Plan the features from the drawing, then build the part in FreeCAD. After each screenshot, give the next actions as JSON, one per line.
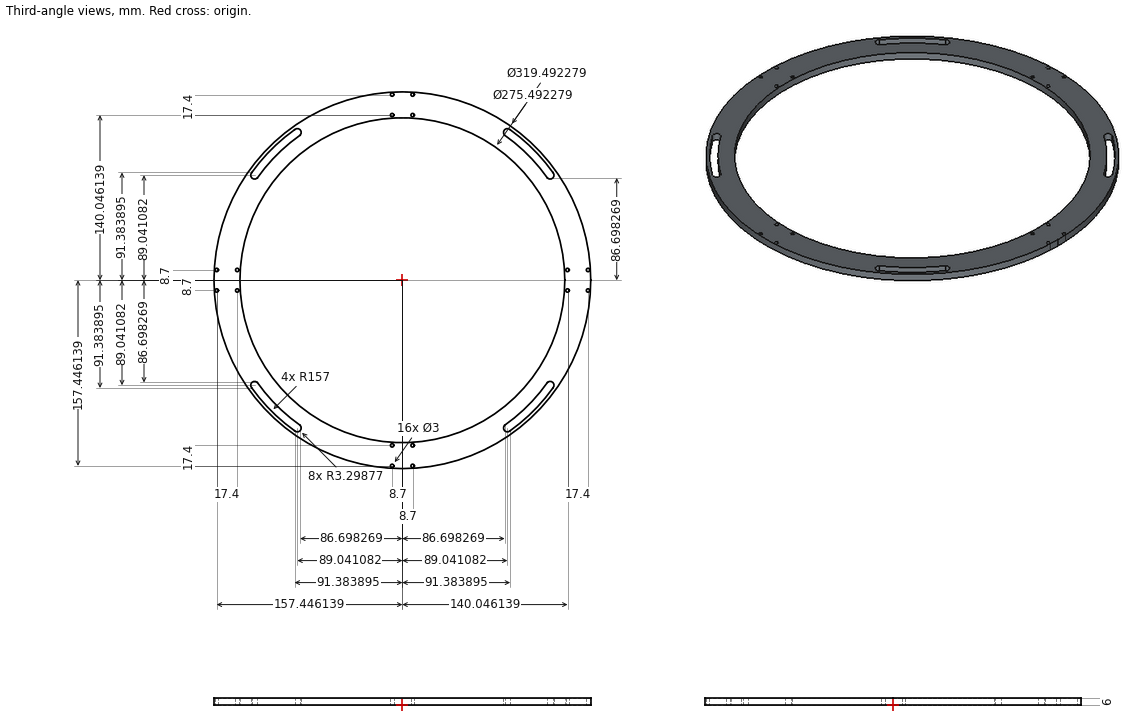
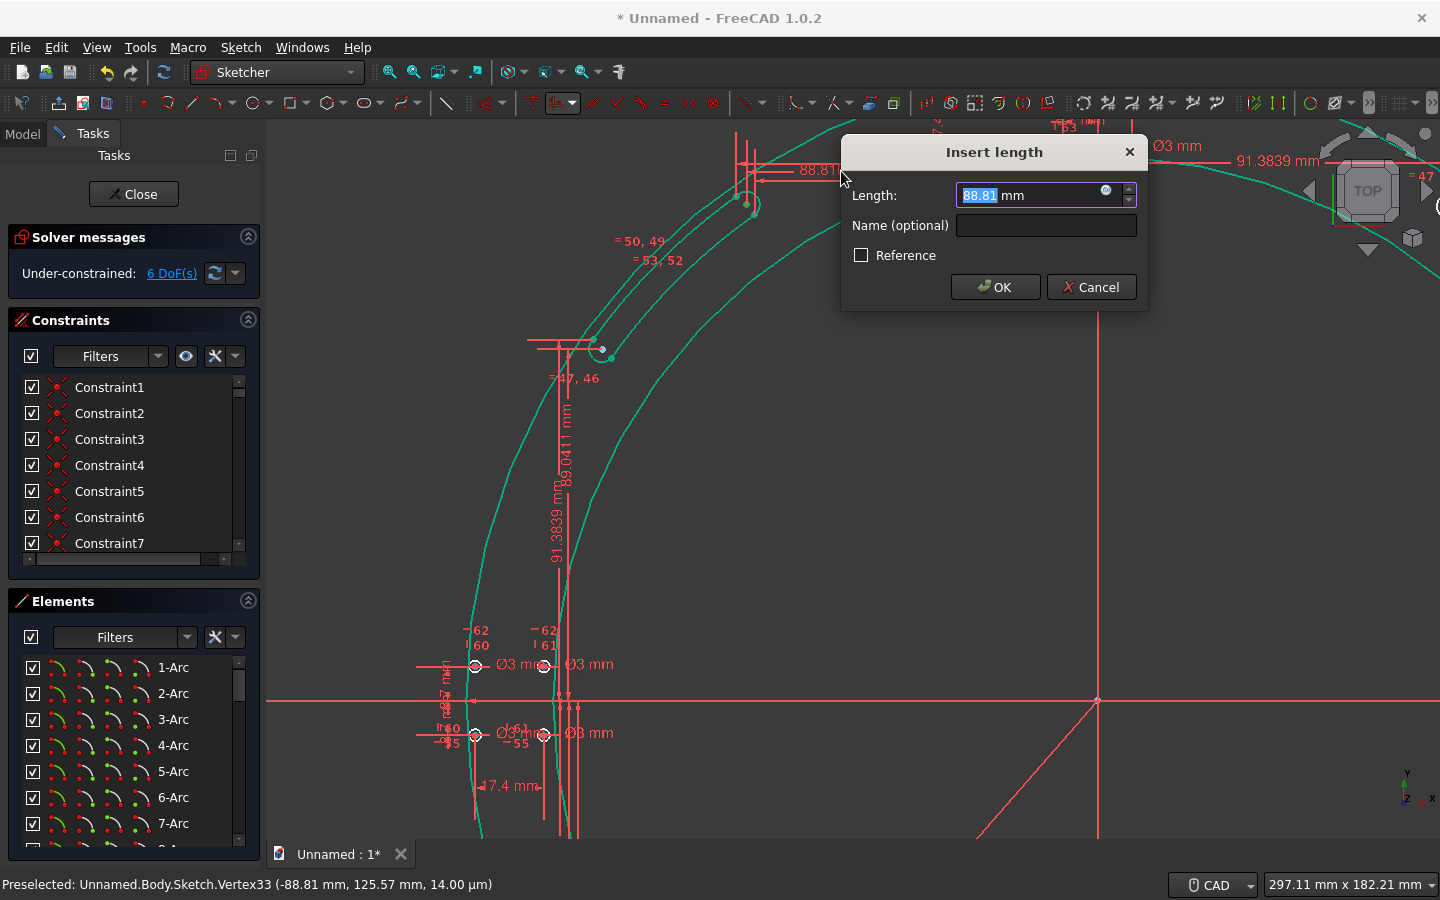
{"action": "type", "text": "89.041082"}
{"action": "key", "text": "Return"}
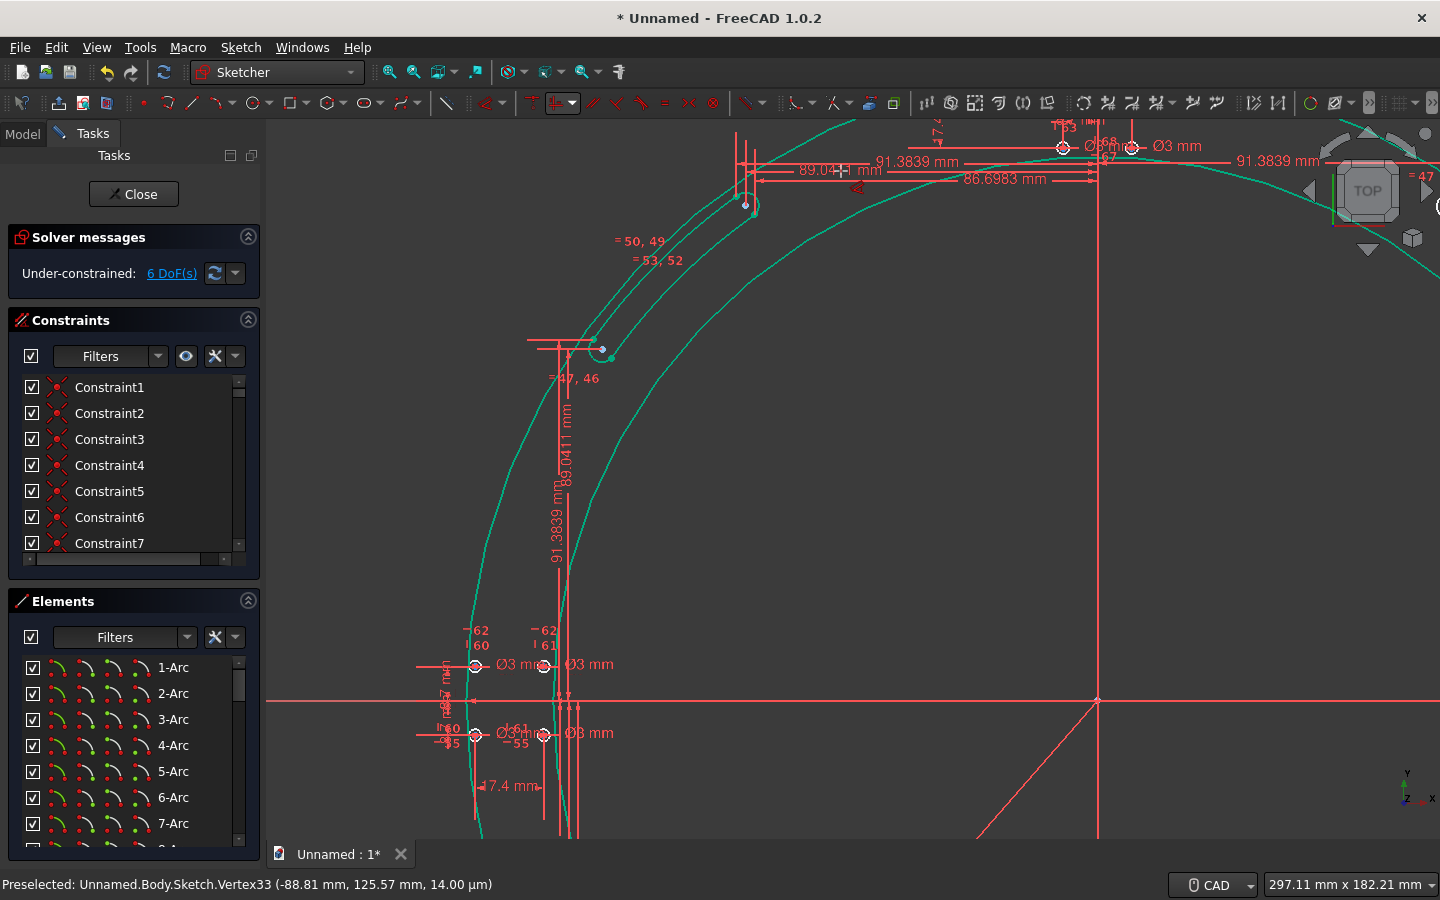
{"action": "scroll", "coordinate": [602, 350], "scroll_direction": "down", "scroll_amount": 5}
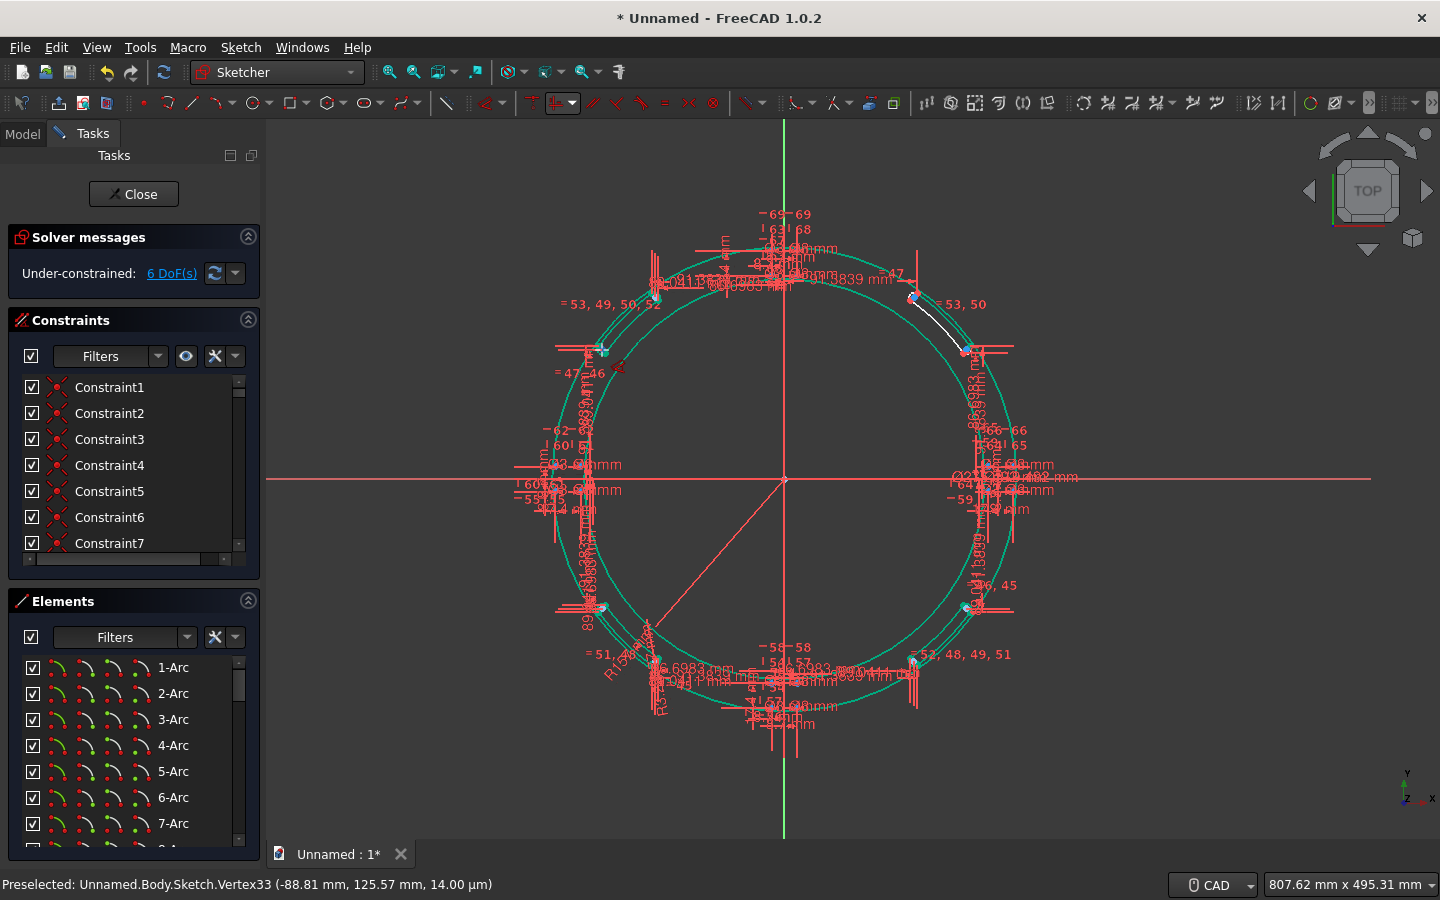
{"action": "scroll", "coordinate": [914, 297], "scroll_direction": "up", "scroll_amount": 5}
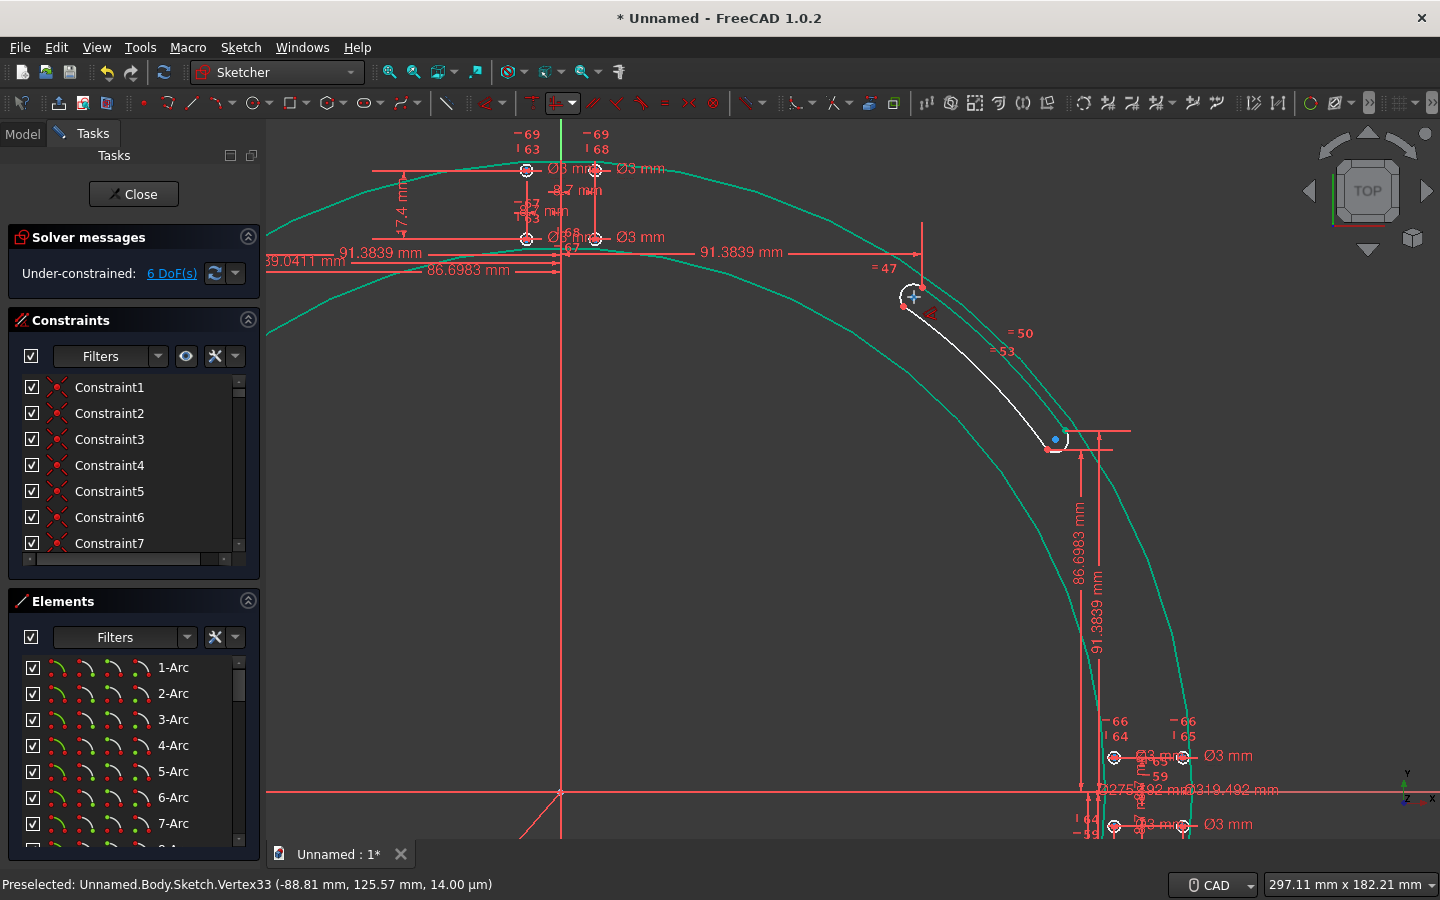
{"action": "left_click", "coordinate": [913, 297]}
{"action": "left_click", "coordinate": [818, 263]}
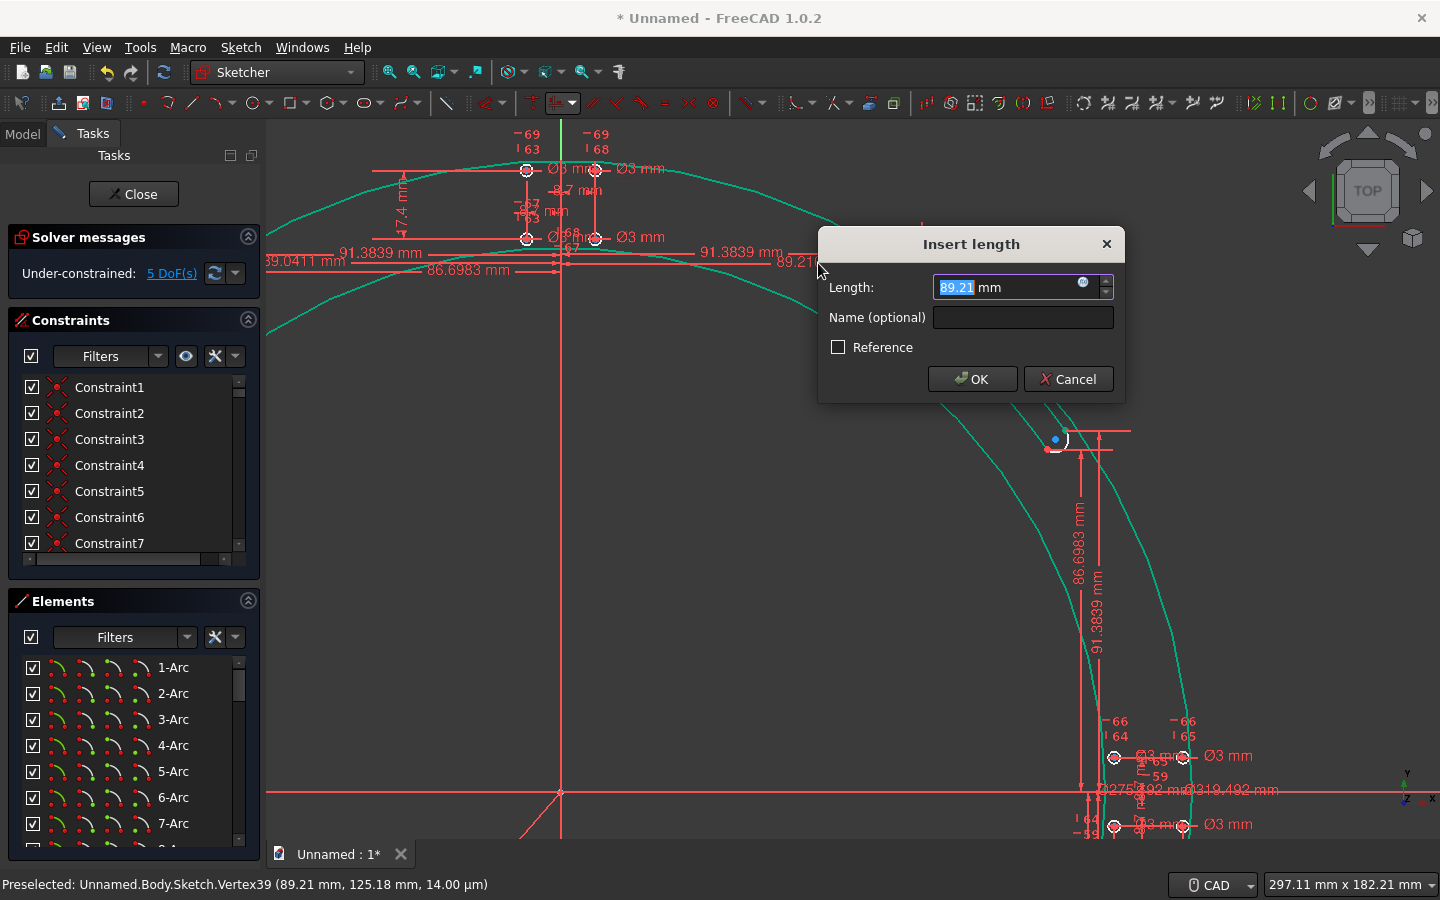
{"action": "type", "text": "89.041082"}
{"action": "key", "text": "Return"}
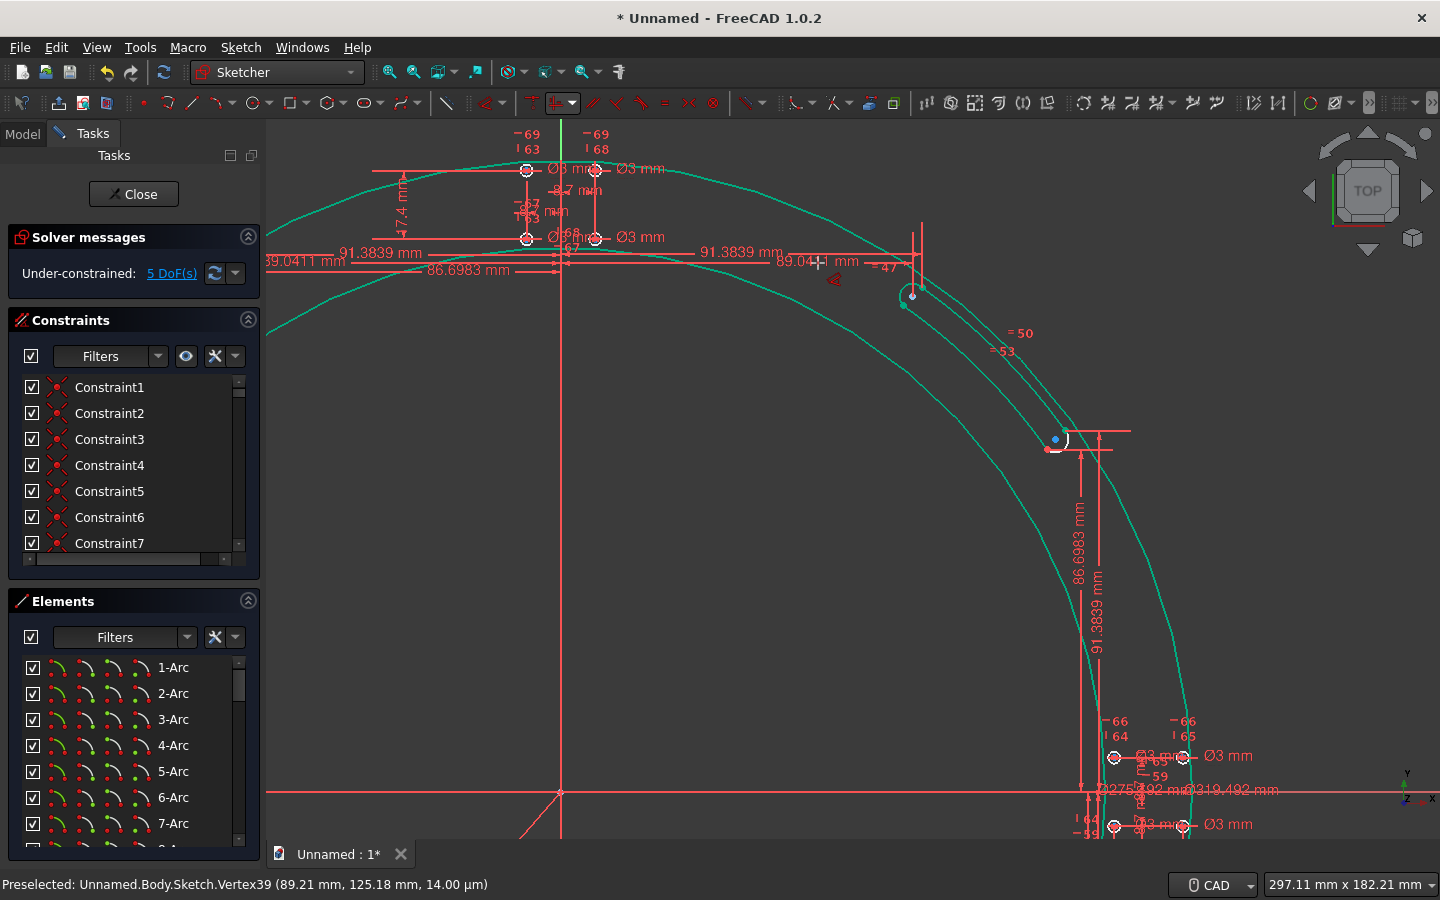
{"action": "left_click", "coordinate": [1055, 439]}
{"action": "left_click", "coordinate": [1089, 492]}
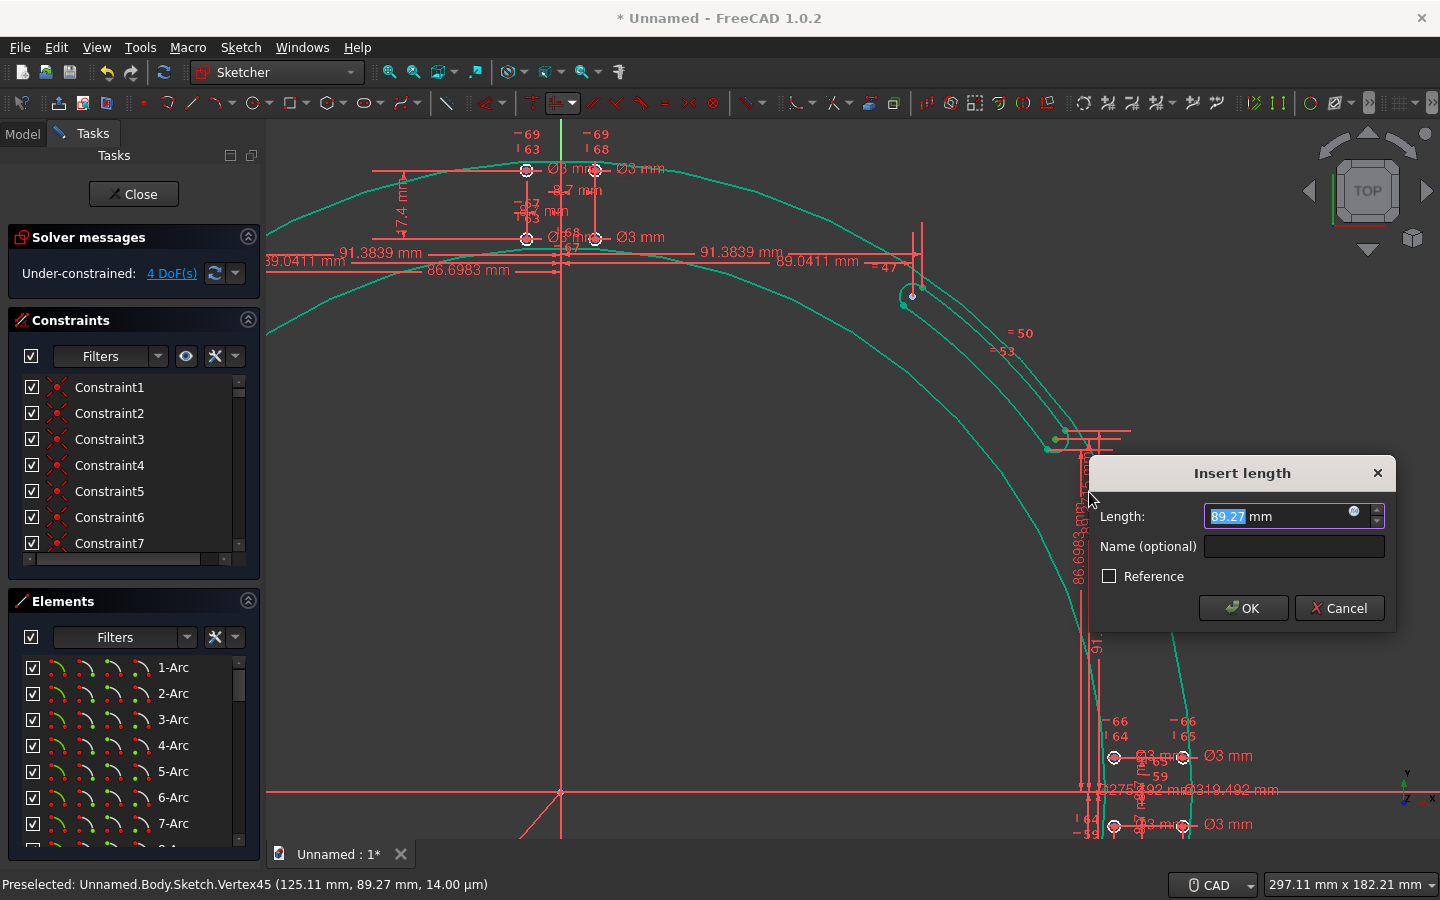
{"action": "type", "text": "89.041082"}
{"action": "key", "text": "Return"}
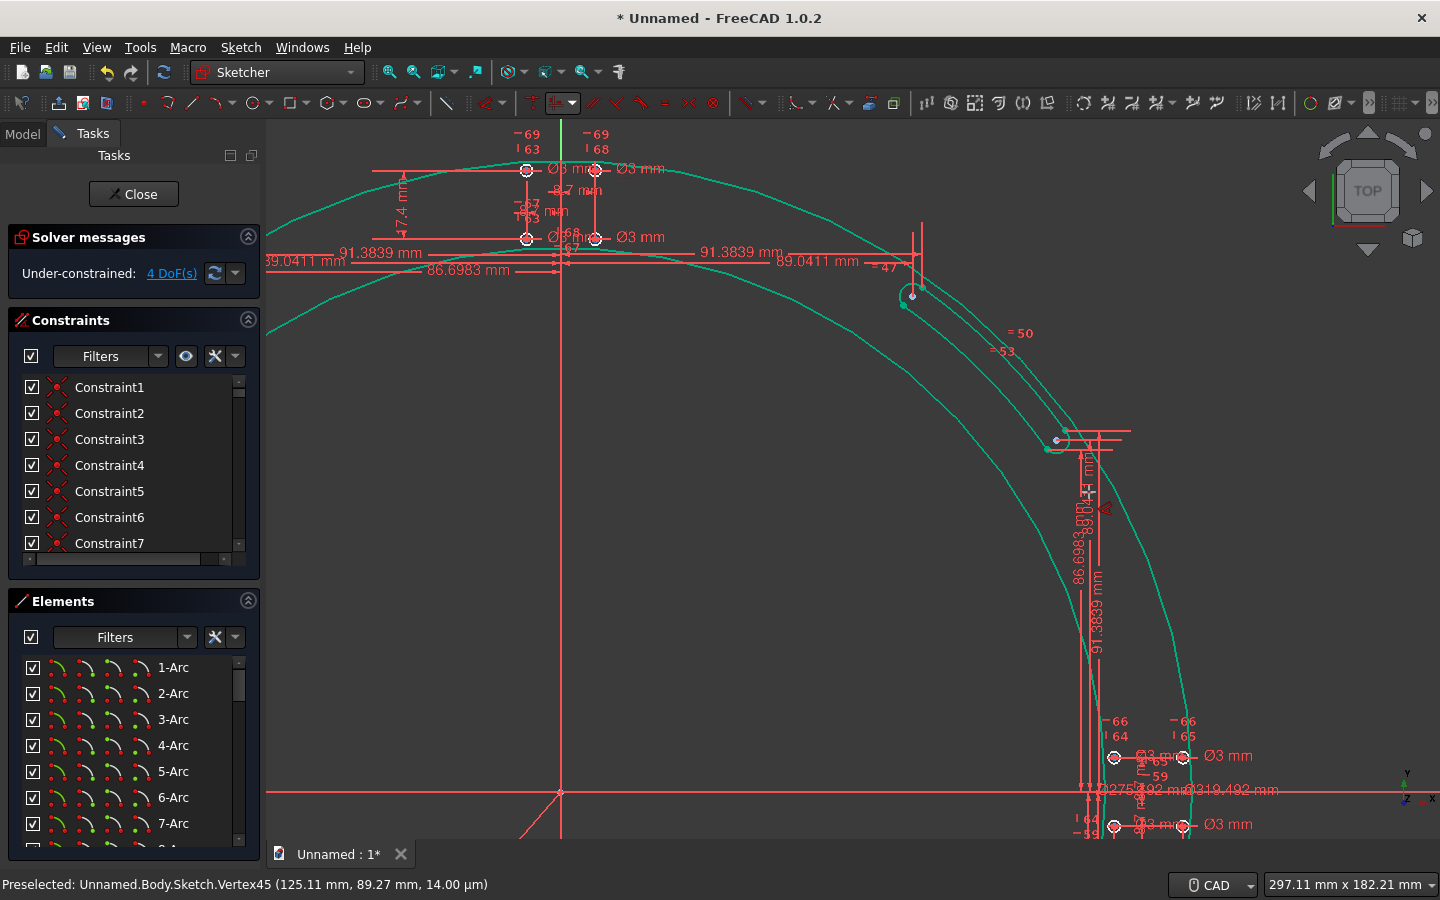
{"action": "scroll", "coordinate": [915, 297], "scroll_direction": "down", "scroll_amount": 5}